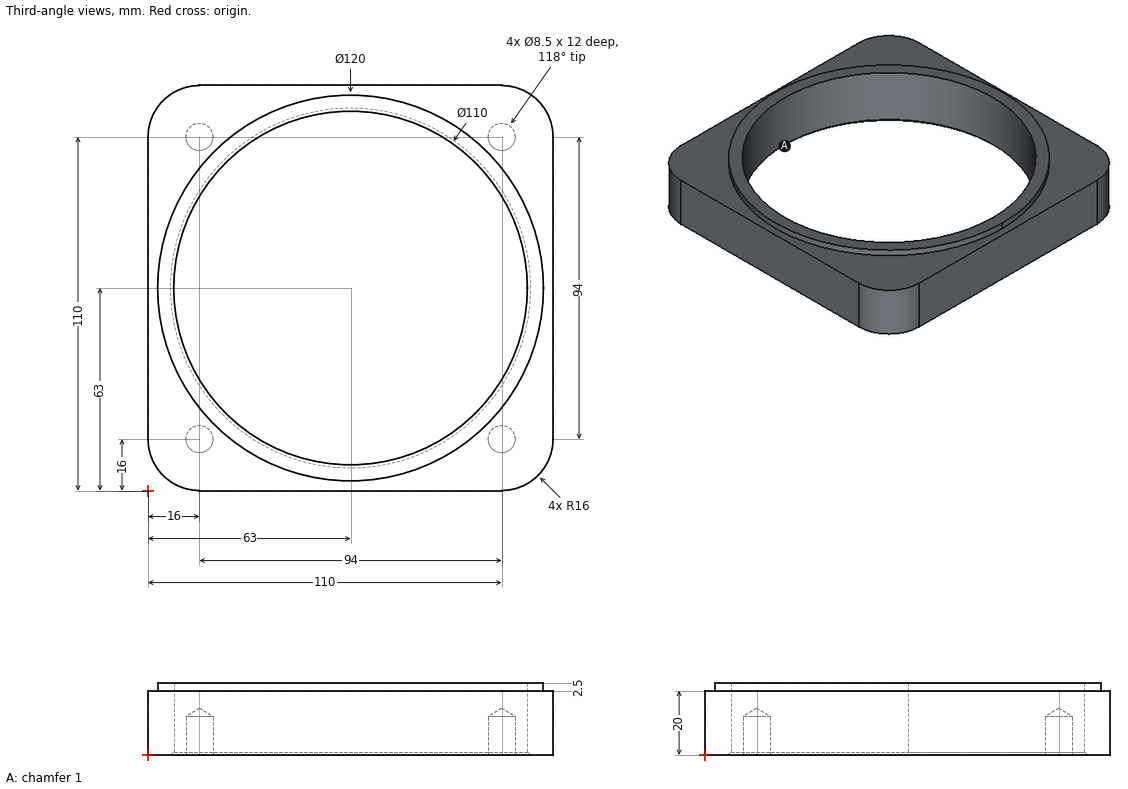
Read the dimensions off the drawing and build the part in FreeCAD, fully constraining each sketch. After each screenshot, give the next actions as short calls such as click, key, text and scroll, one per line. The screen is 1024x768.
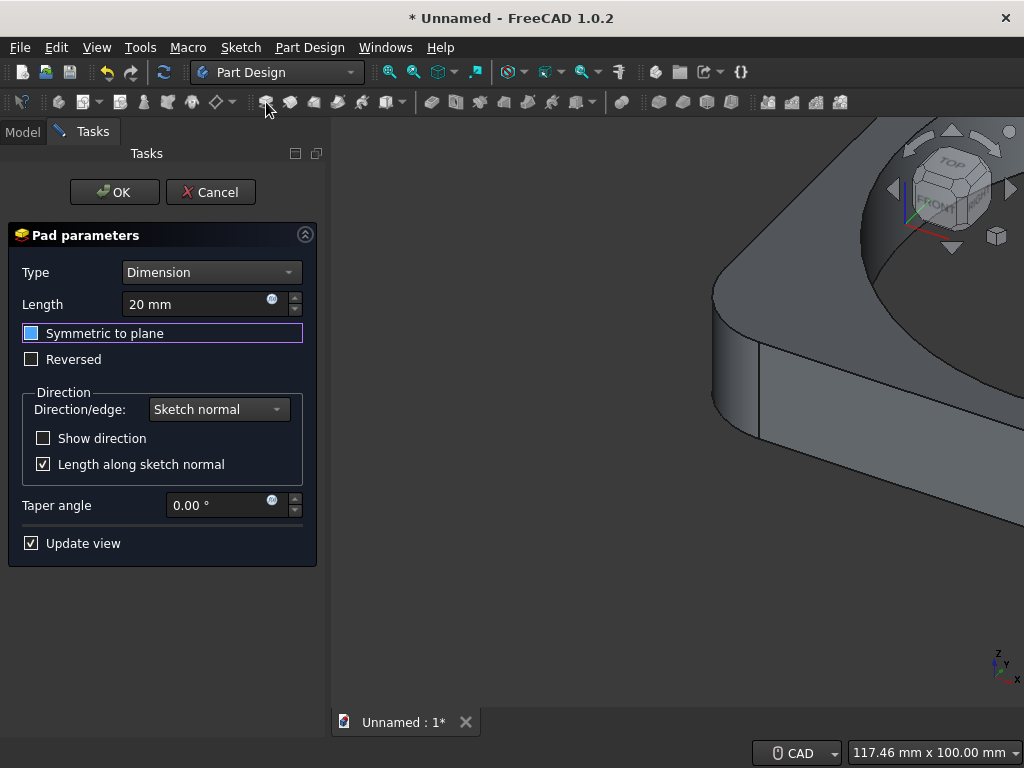
click(115, 192)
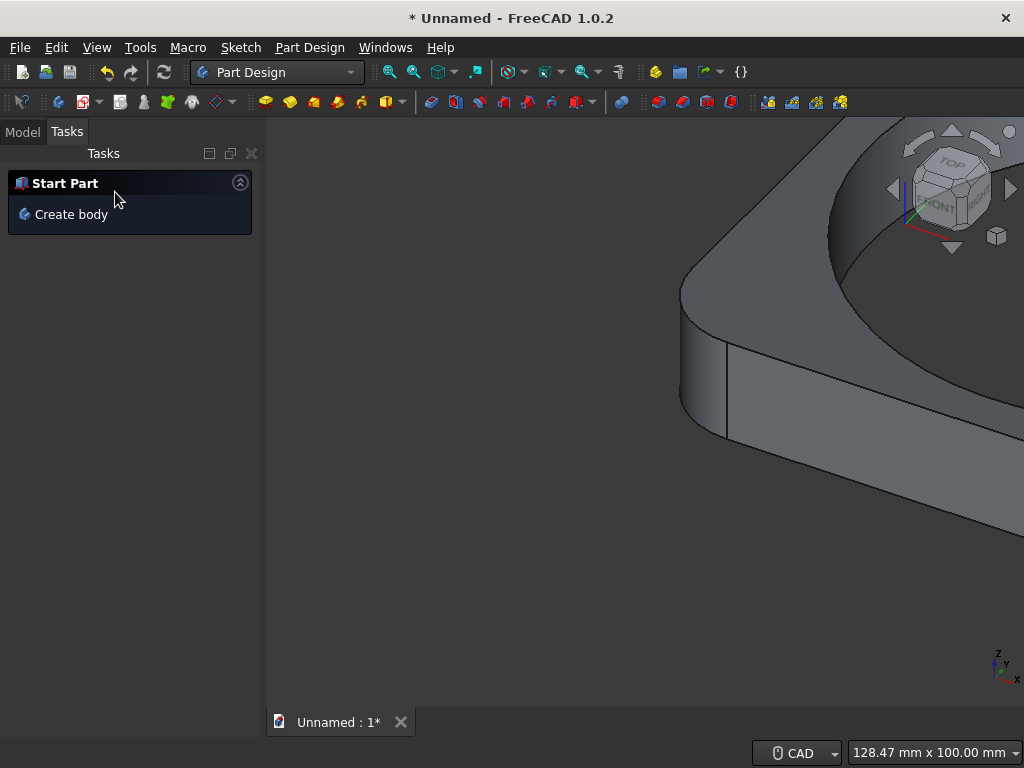
click(390, 72)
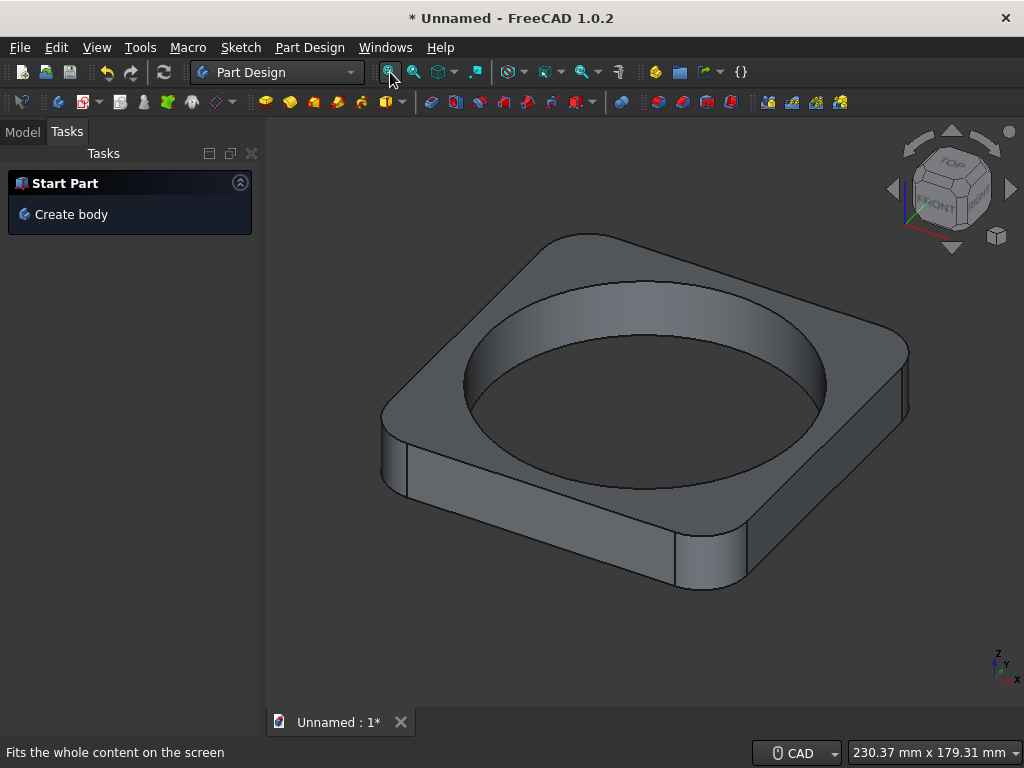
click(858, 376)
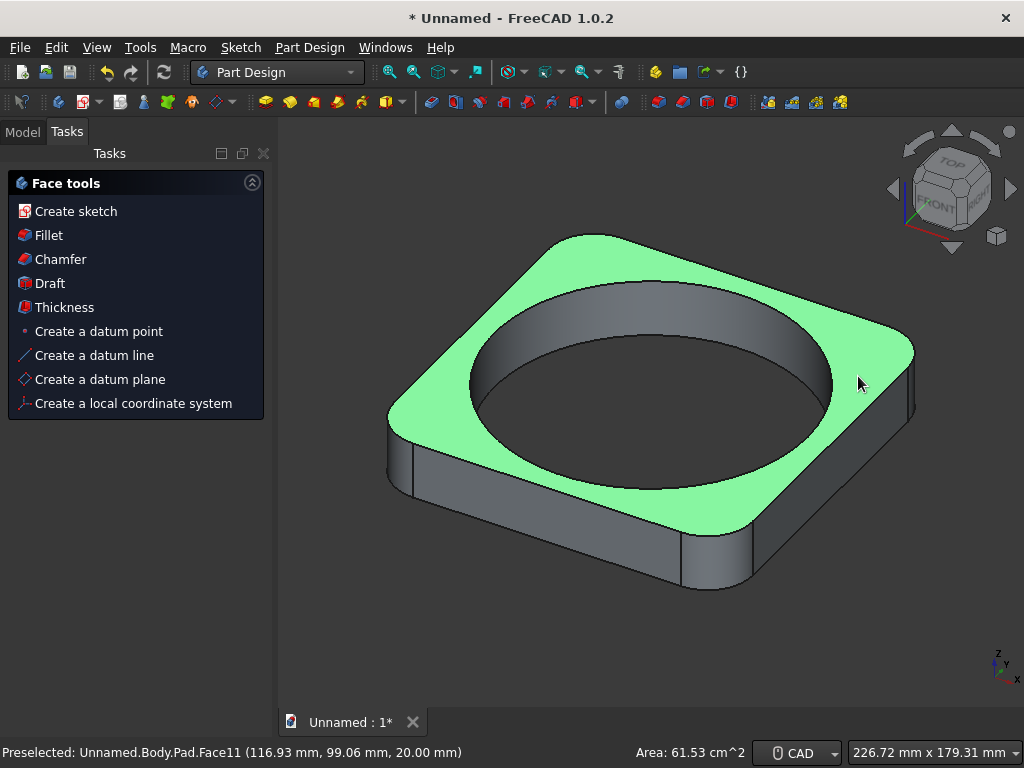
click(84, 102)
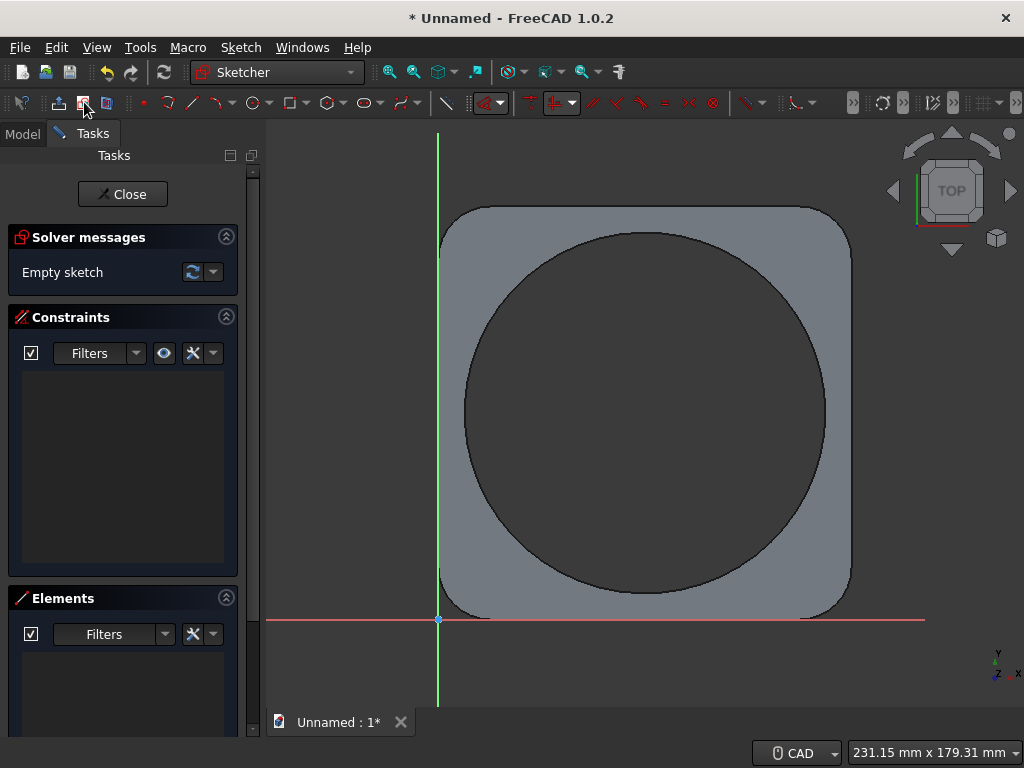
scroll(294, 391, down, 1)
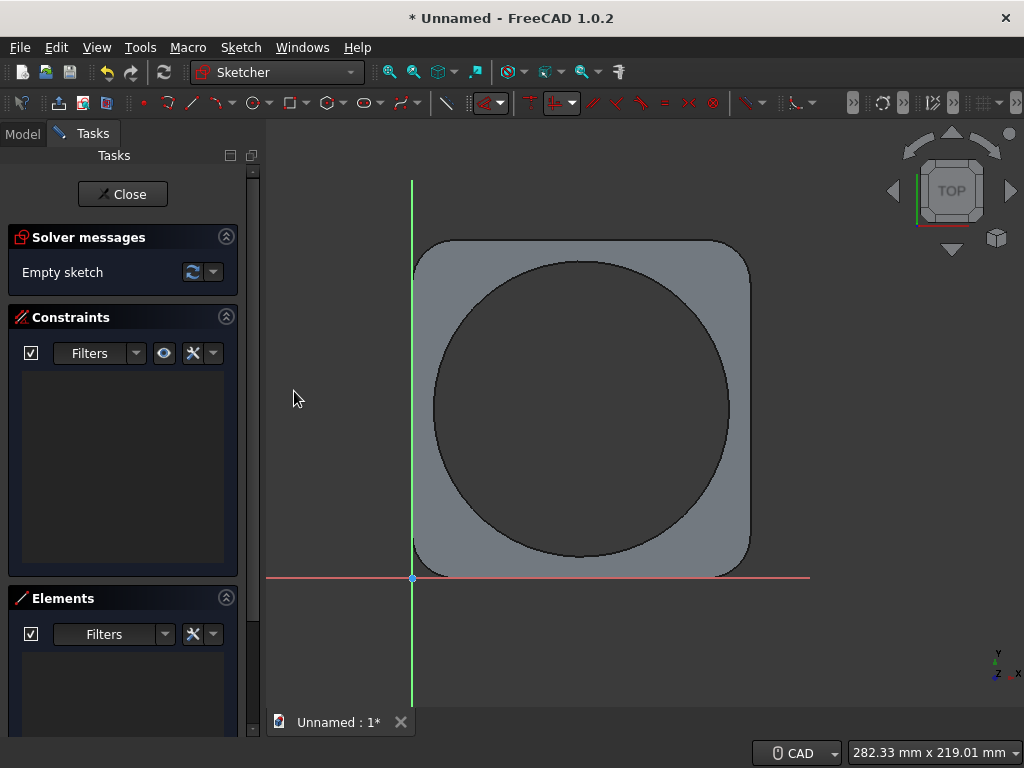
click(254, 104)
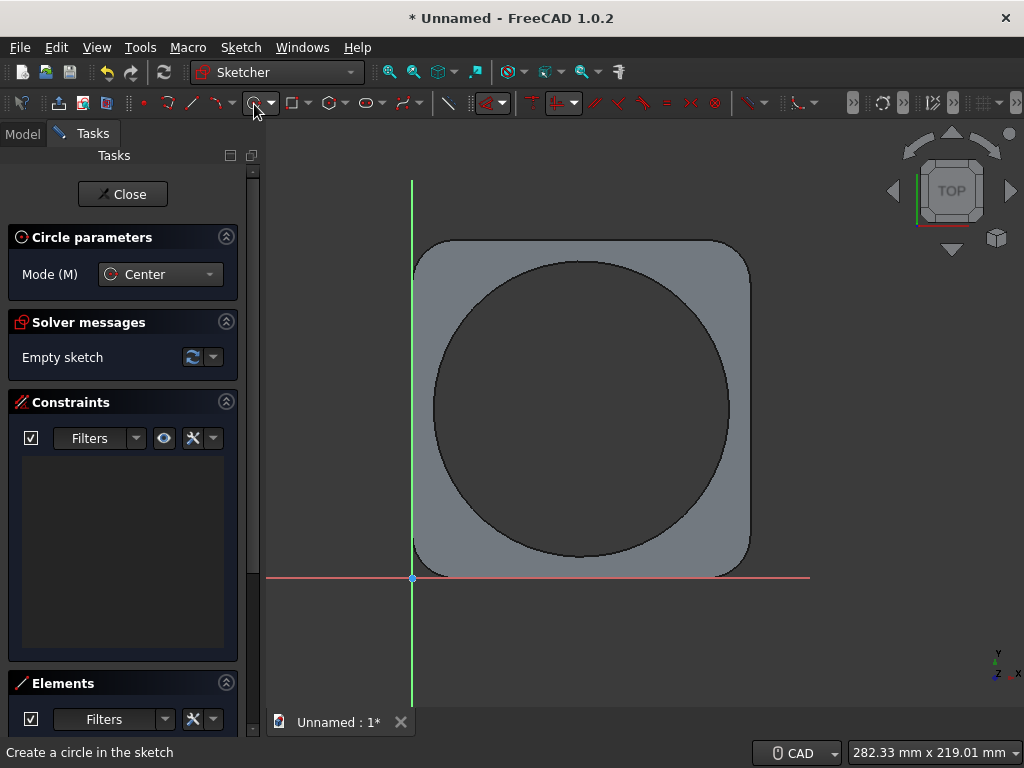
click(581, 409)
move(695, 295)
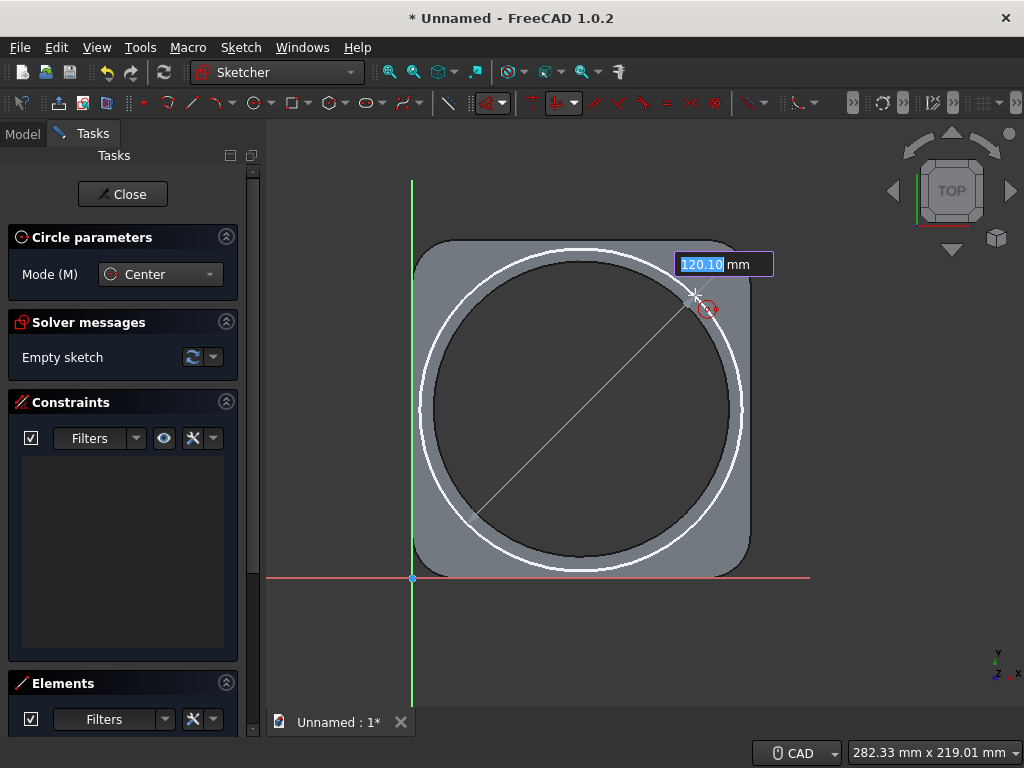
text(120)
key(Return)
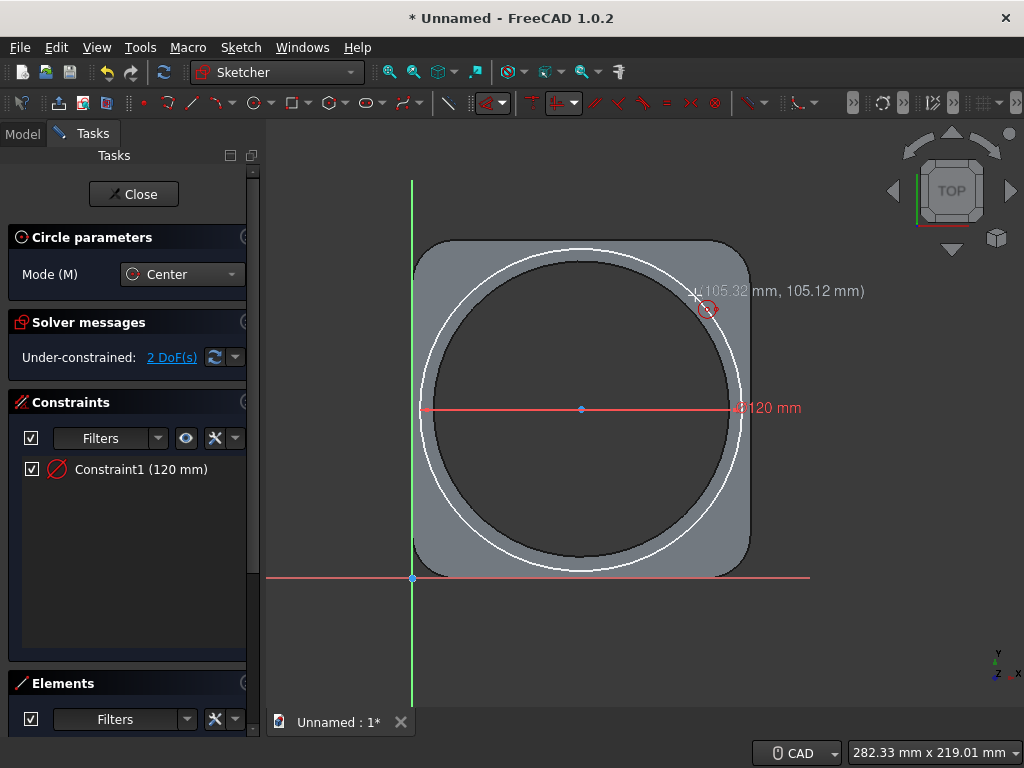
click(581, 410)
move(686, 305)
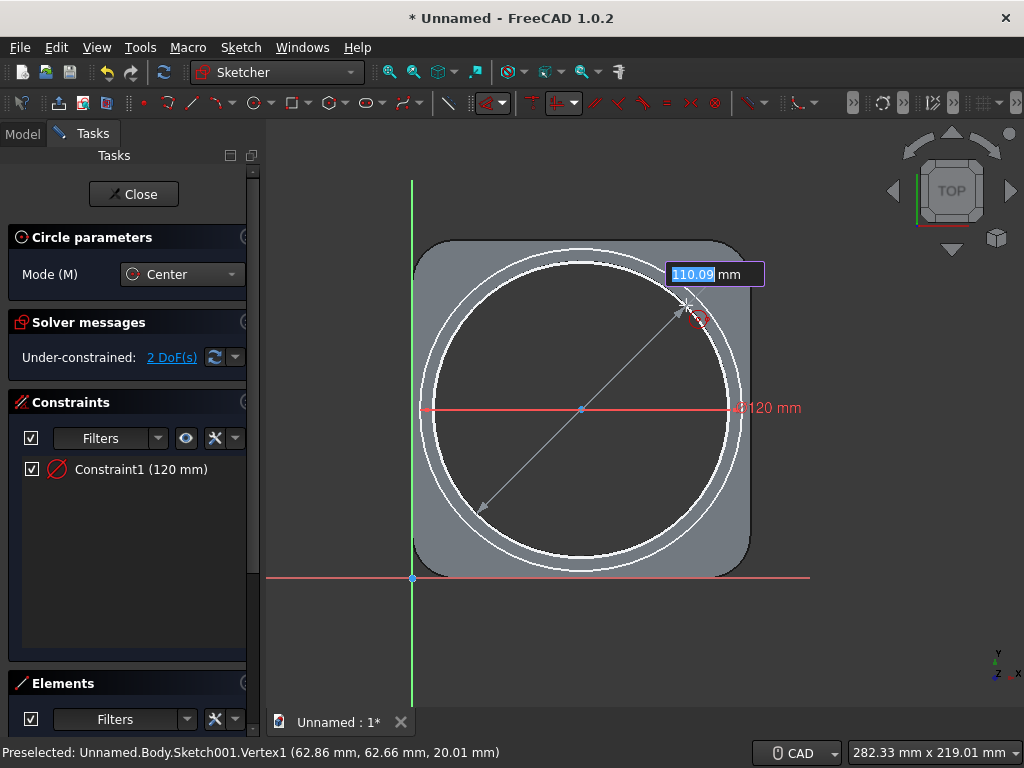
text(110)
key(Return)
key(Escape)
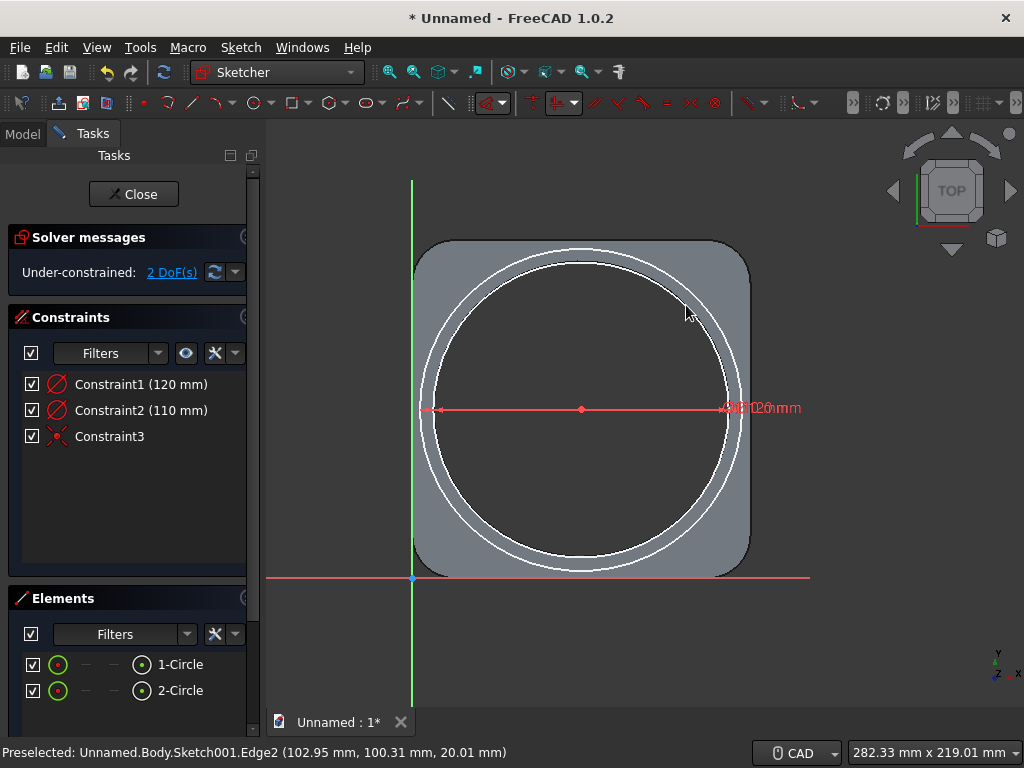
click(581, 410)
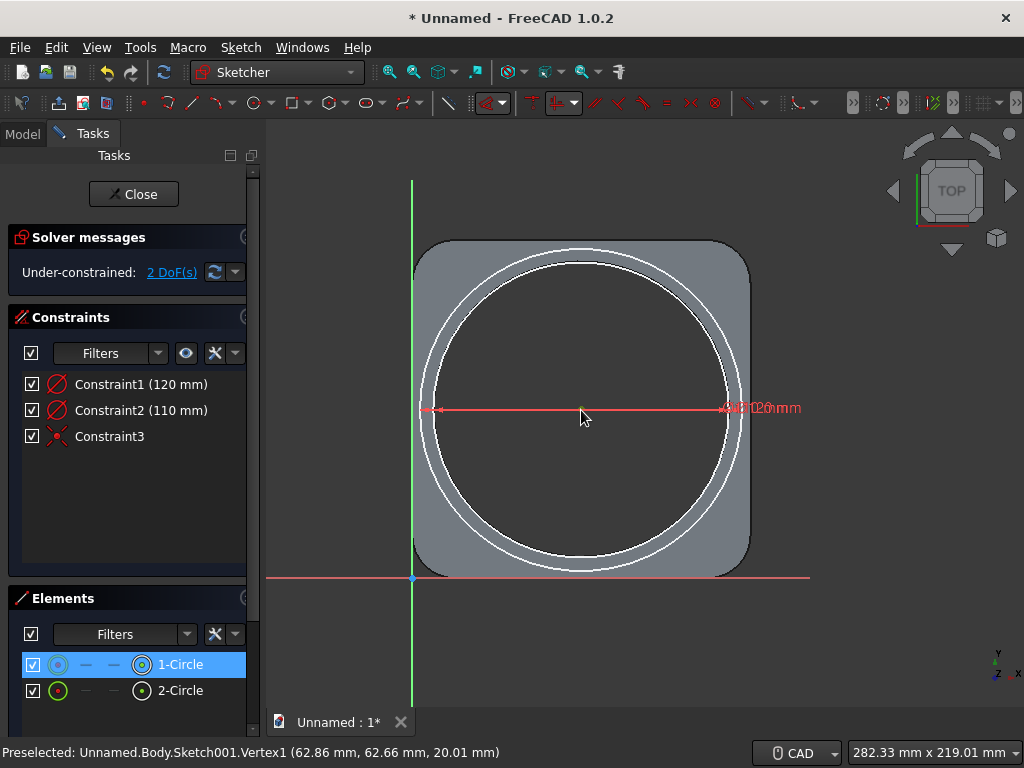
key(l)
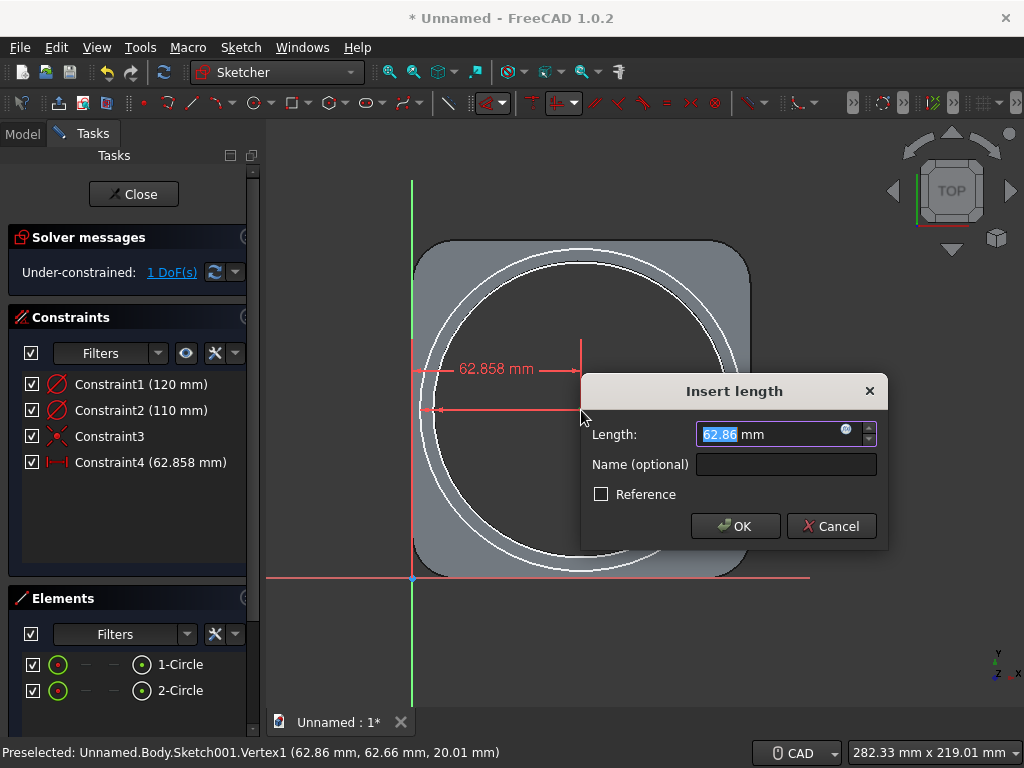
text(63)
key(Return)